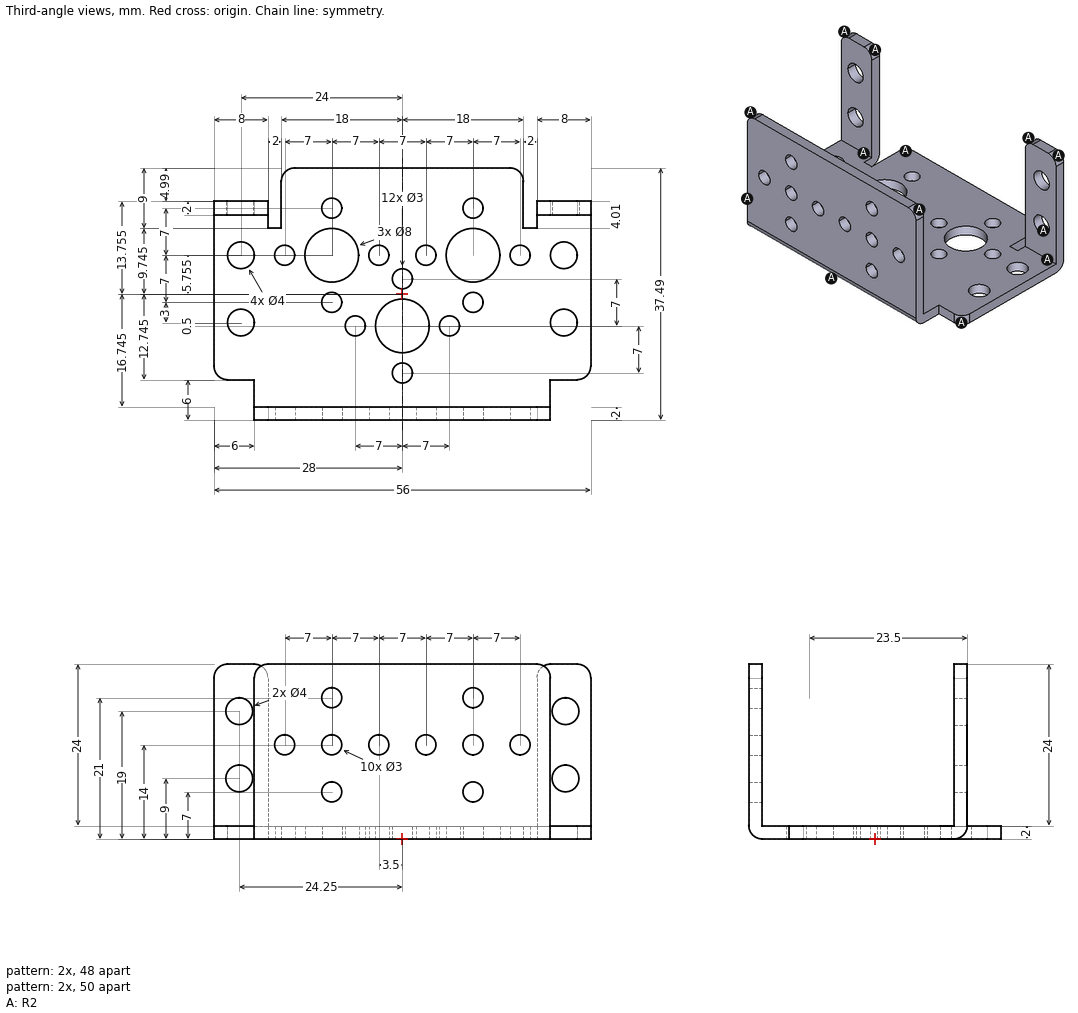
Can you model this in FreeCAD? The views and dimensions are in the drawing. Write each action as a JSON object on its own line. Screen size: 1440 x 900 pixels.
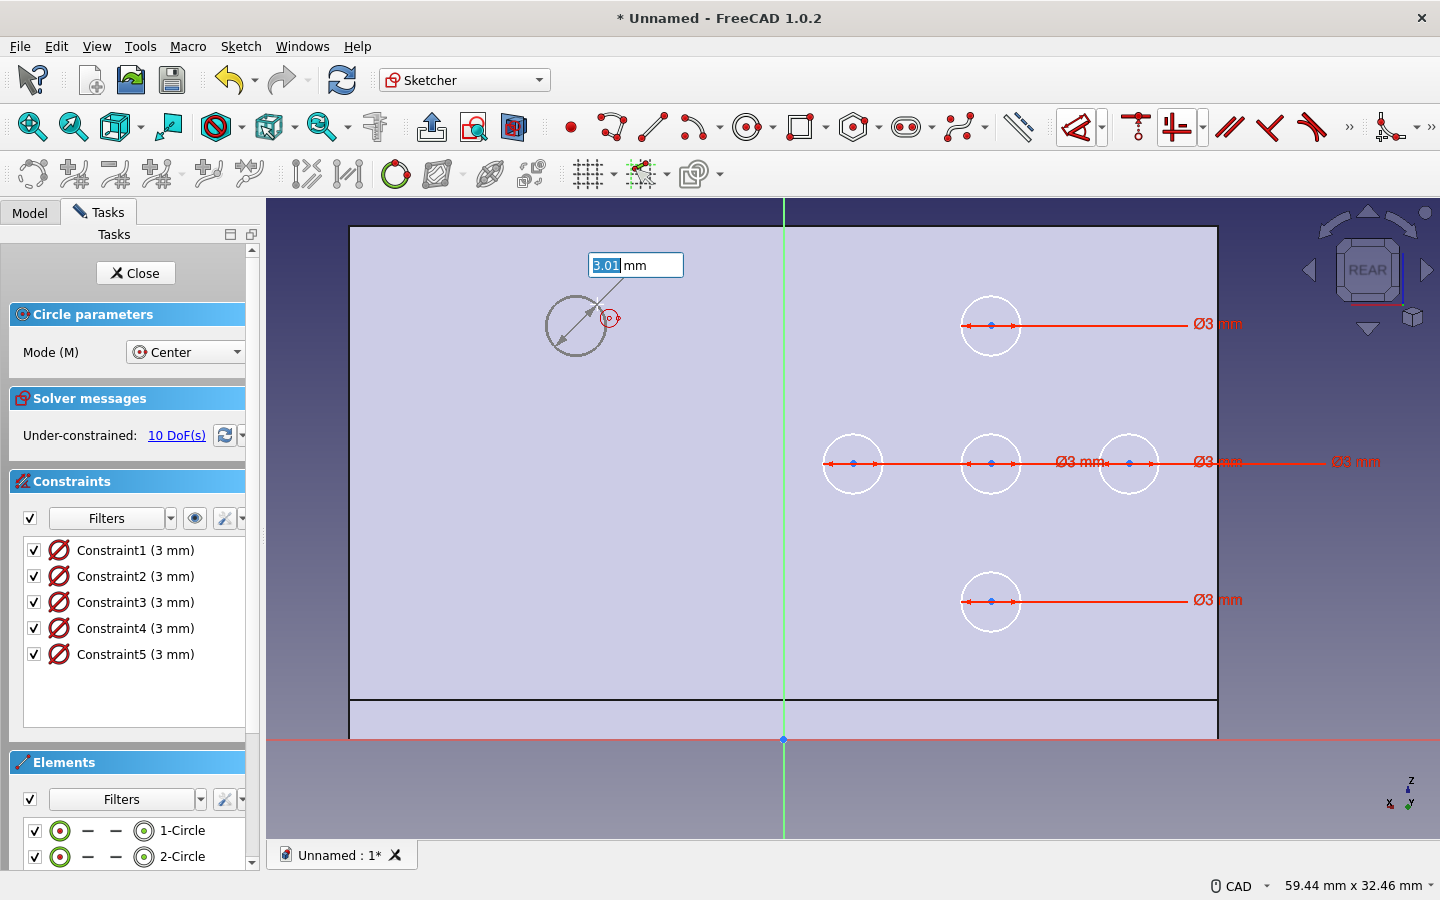
{"action": "type", "text": "3"}
{"action": "key", "text": "Return"}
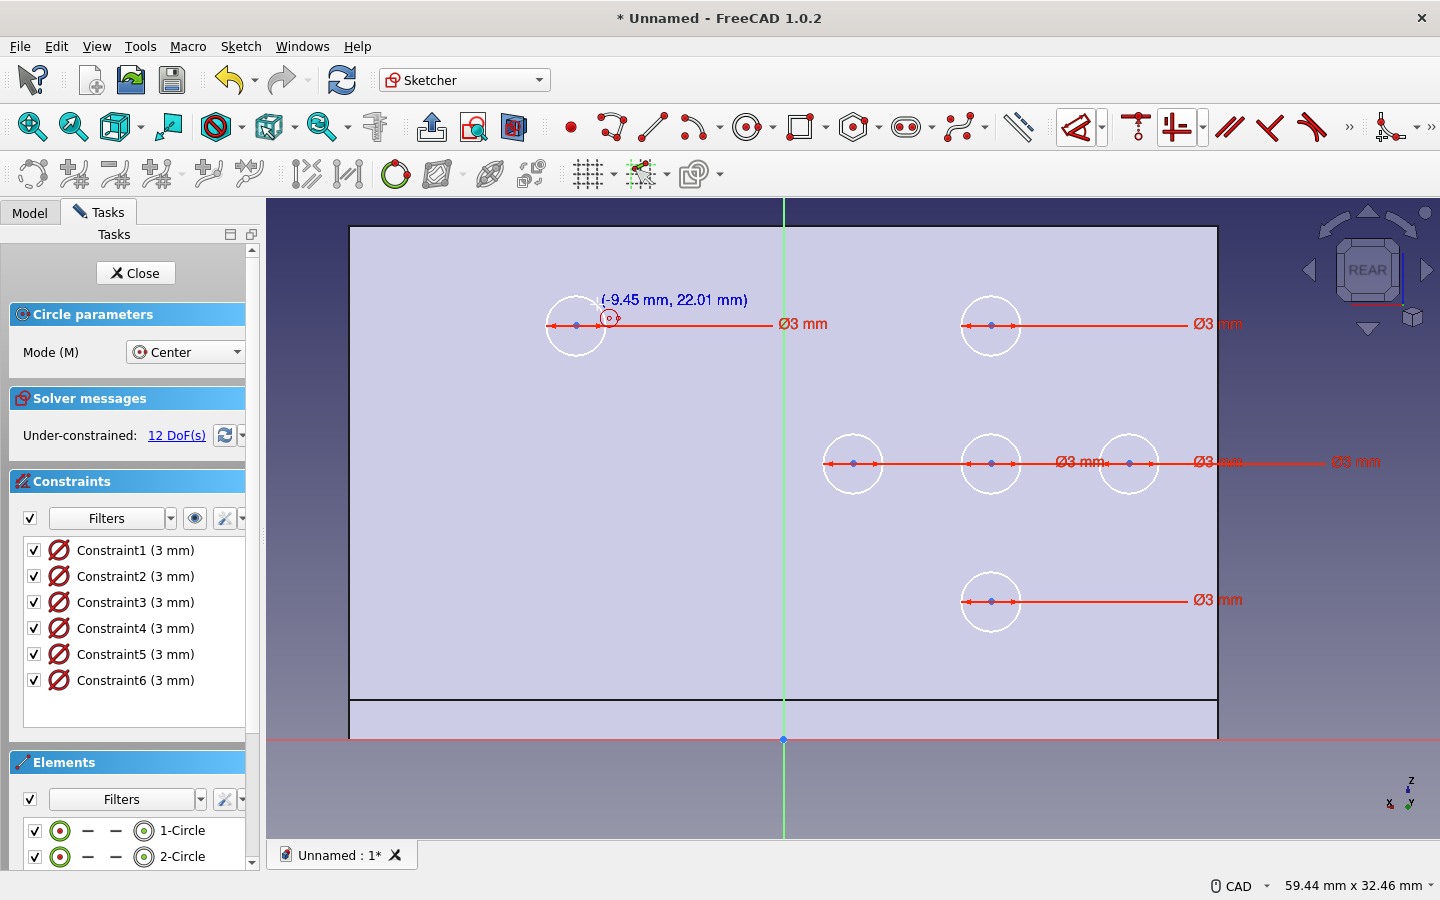
{"action": "left_click", "coordinate": [715, 463]}
{"action": "mouse_move", "coordinate": [736, 442]}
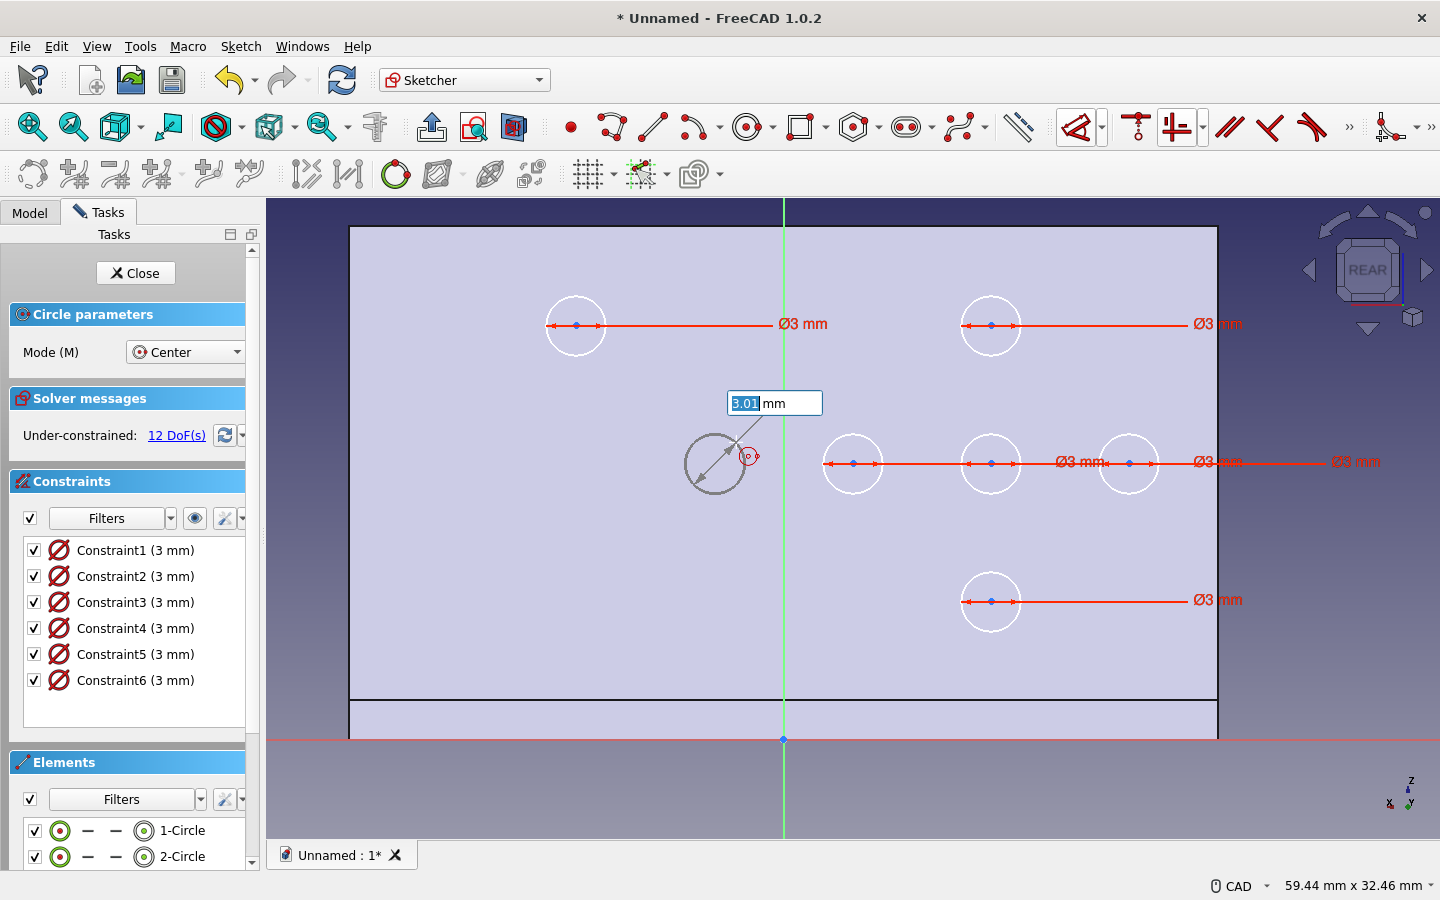
{"action": "type", "text": "3"}
{"action": "key", "text": "Return"}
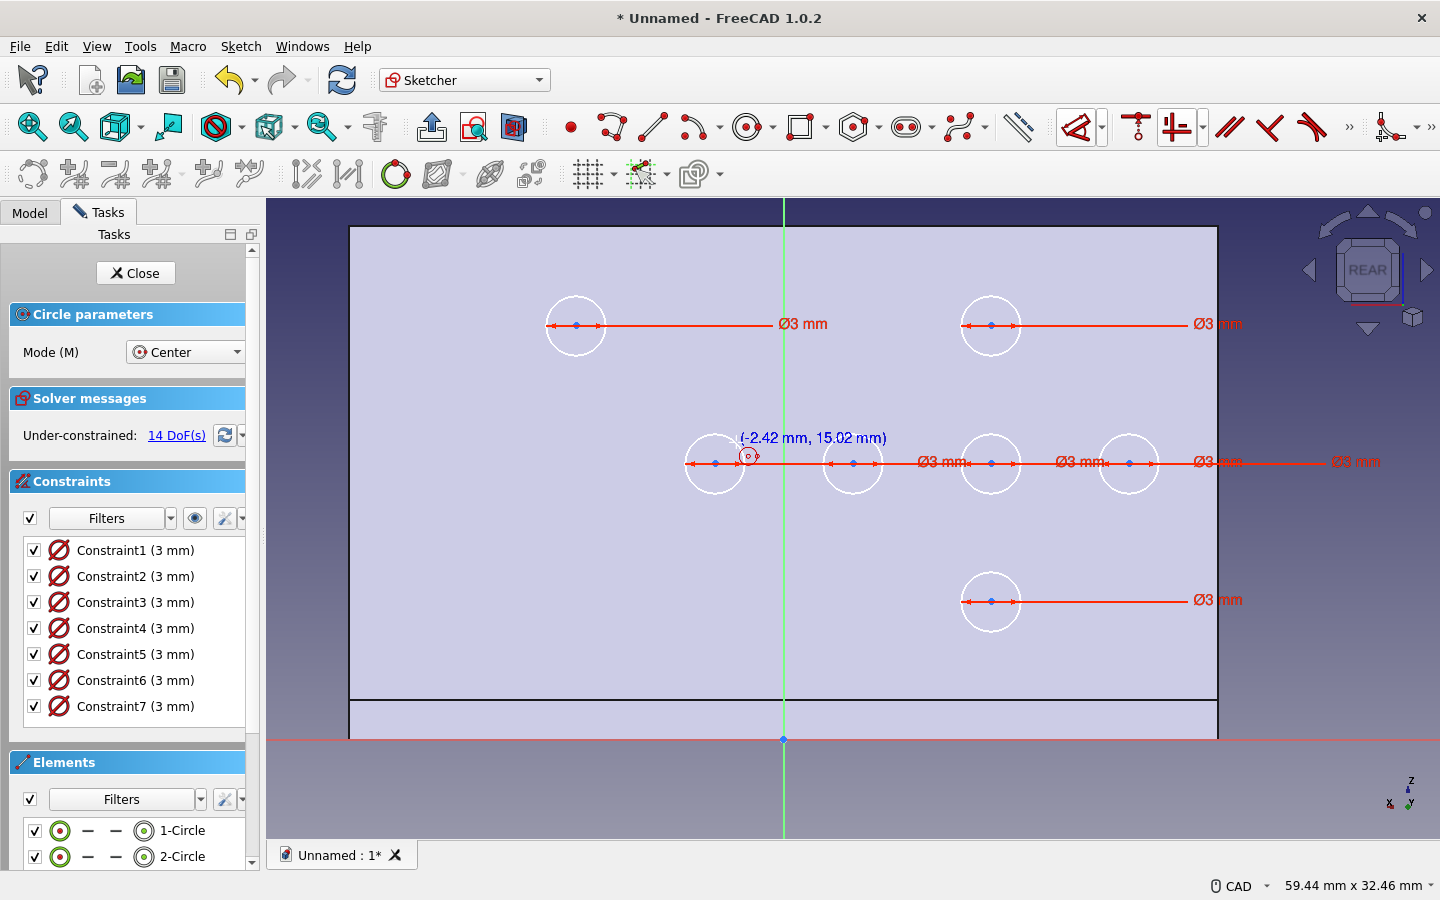
{"action": "left_click", "coordinate": [576, 601]}
{"action": "mouse_move", "coordinate": [597, 580]}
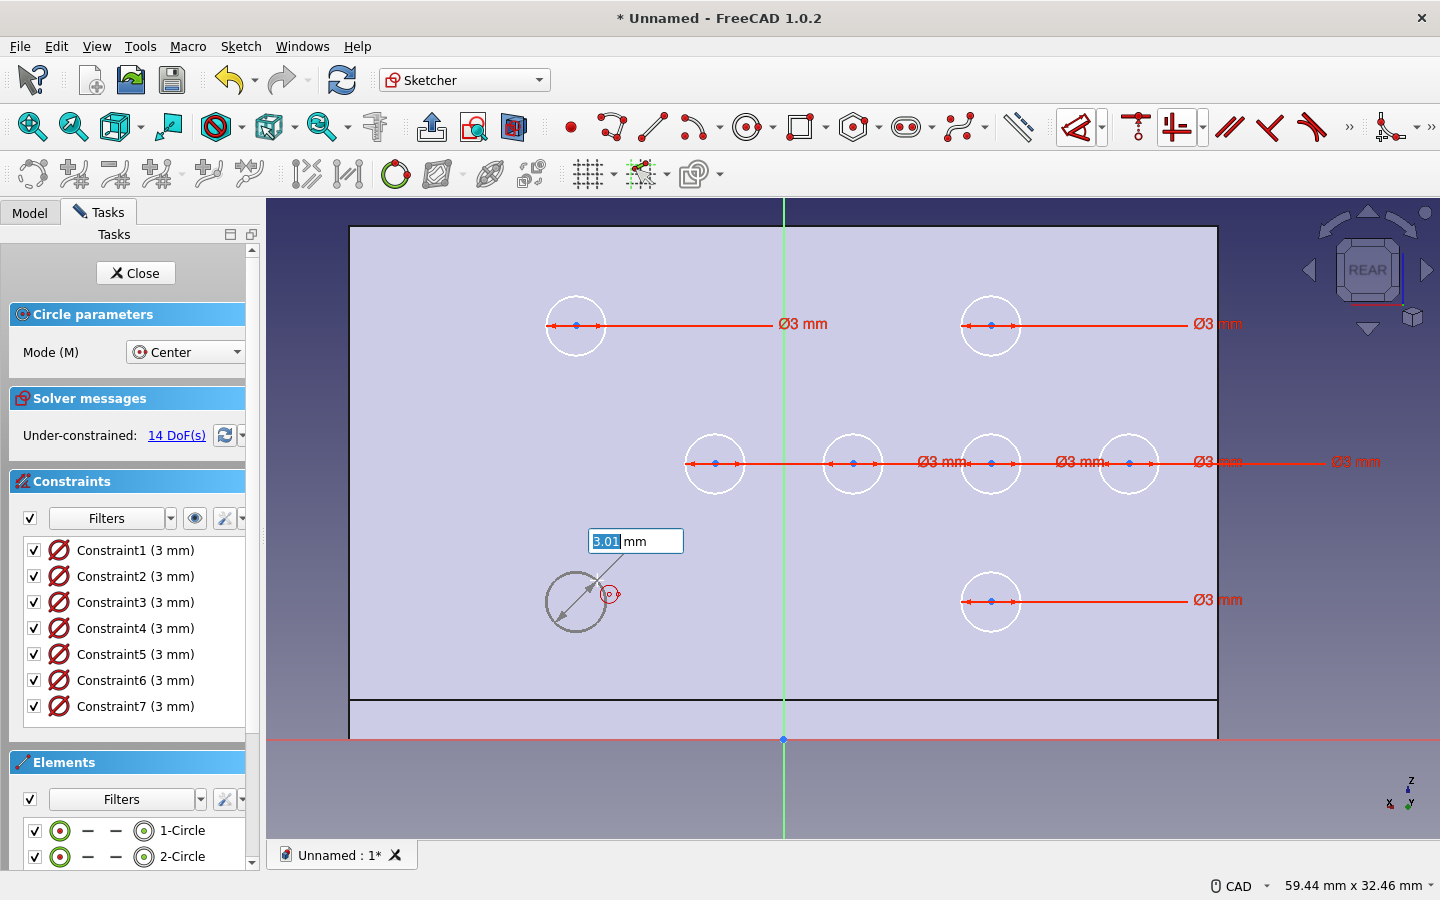
{"action": "type", "text": "3"}
{"action": "key", "text": "Return"}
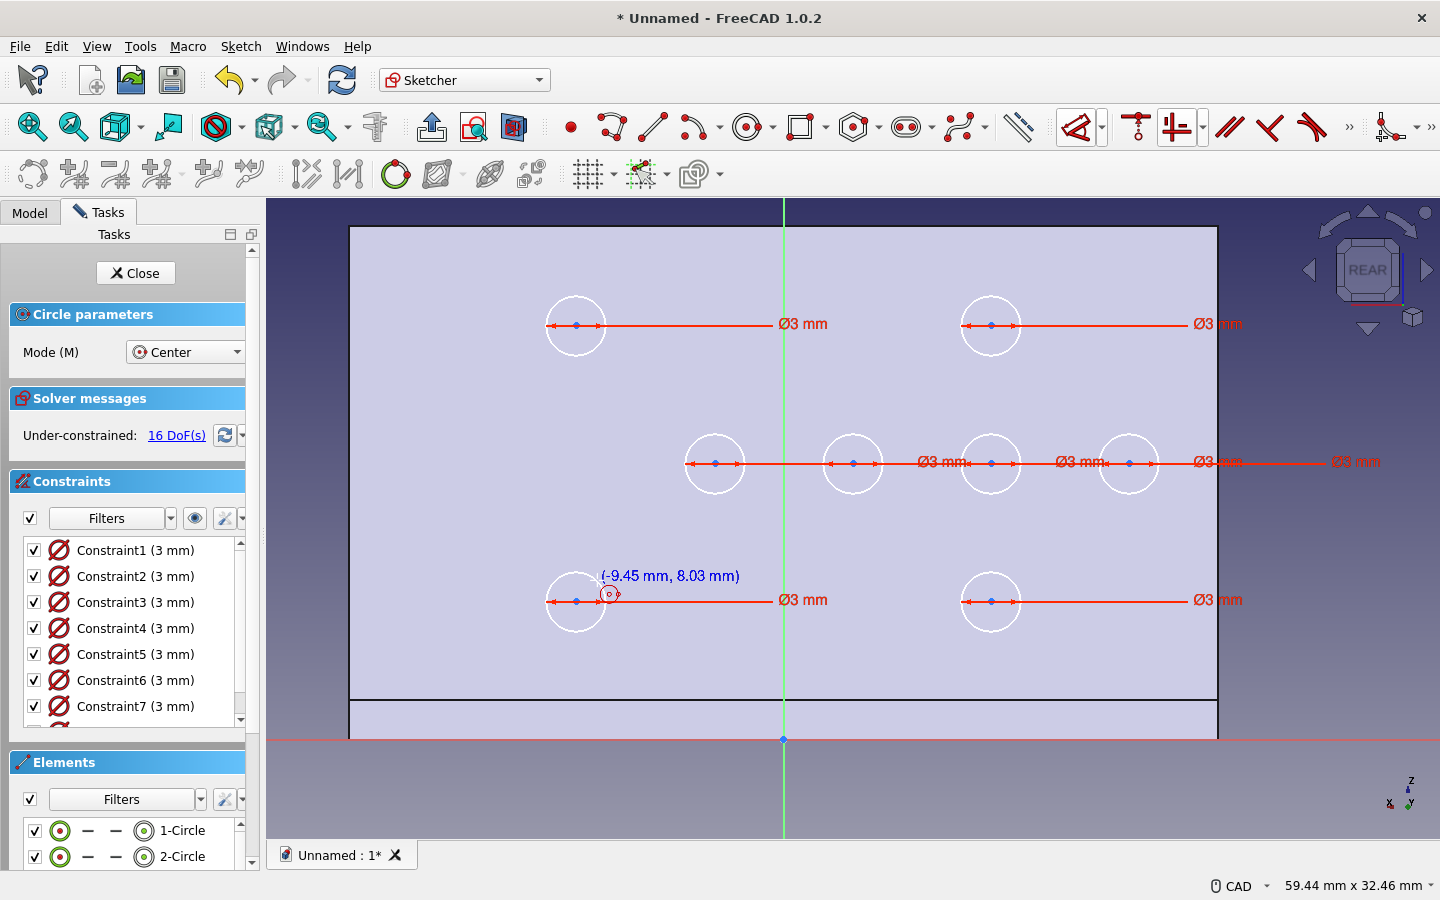
{"action": "left_click", "coordinate": [576, 463]}
{"action": "mouse_move", "coordinate": [597, 442]}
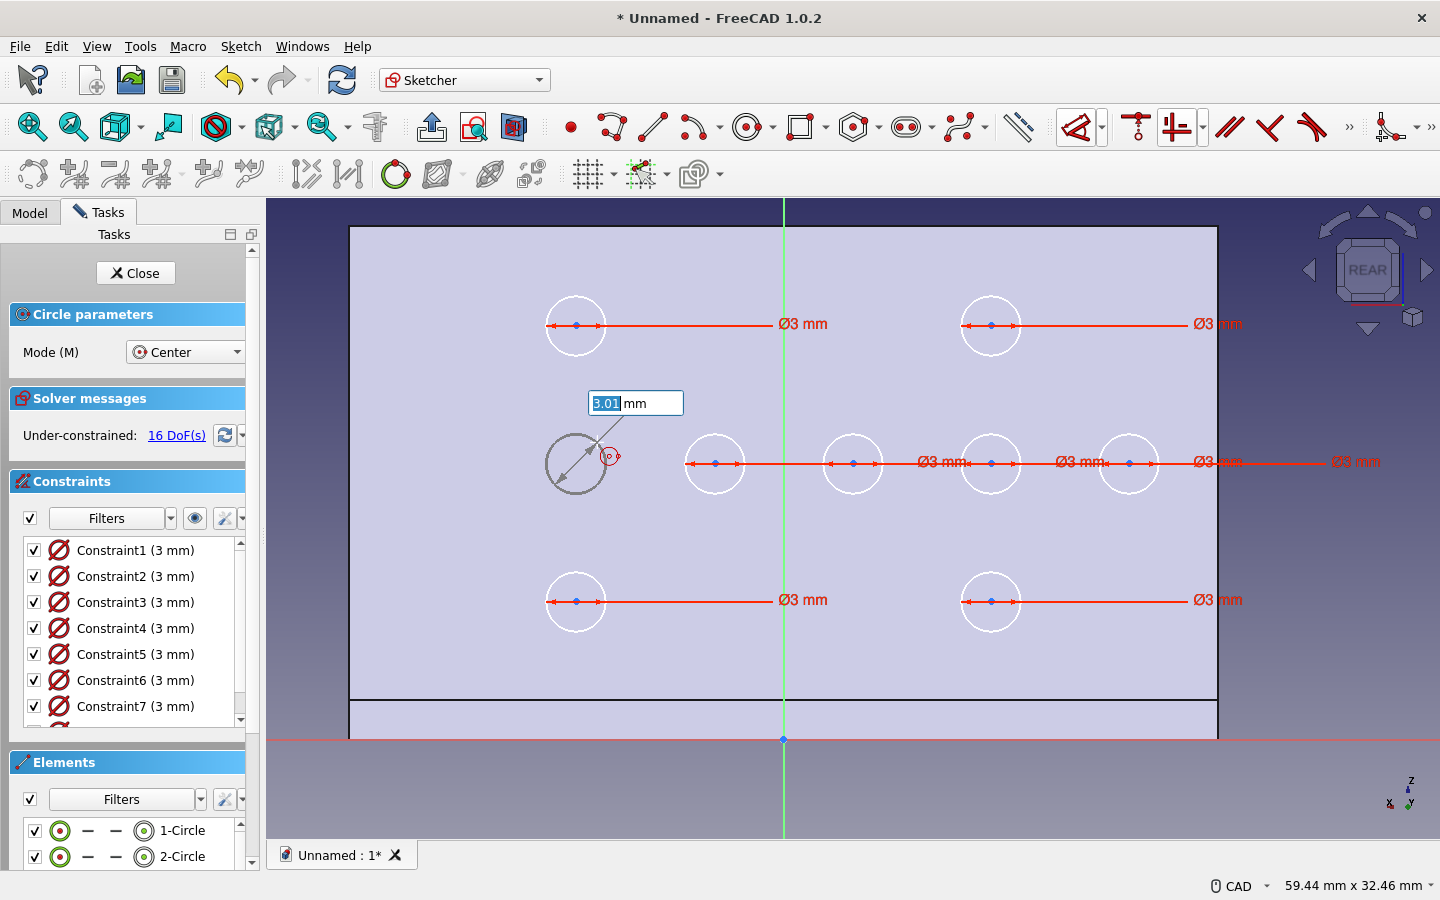
{"action": "type", "text": "3"}
{"action": "key", "text": "Return"}